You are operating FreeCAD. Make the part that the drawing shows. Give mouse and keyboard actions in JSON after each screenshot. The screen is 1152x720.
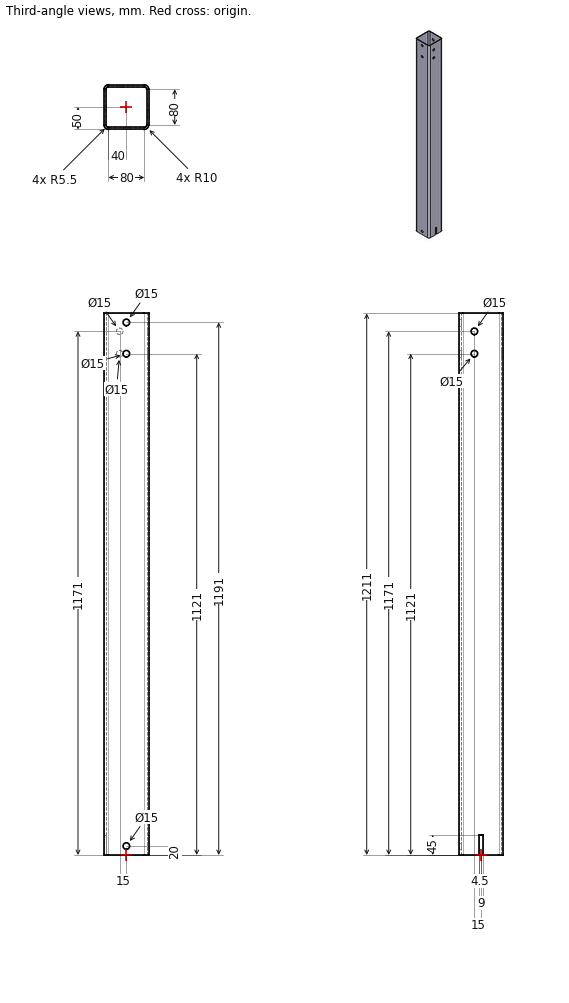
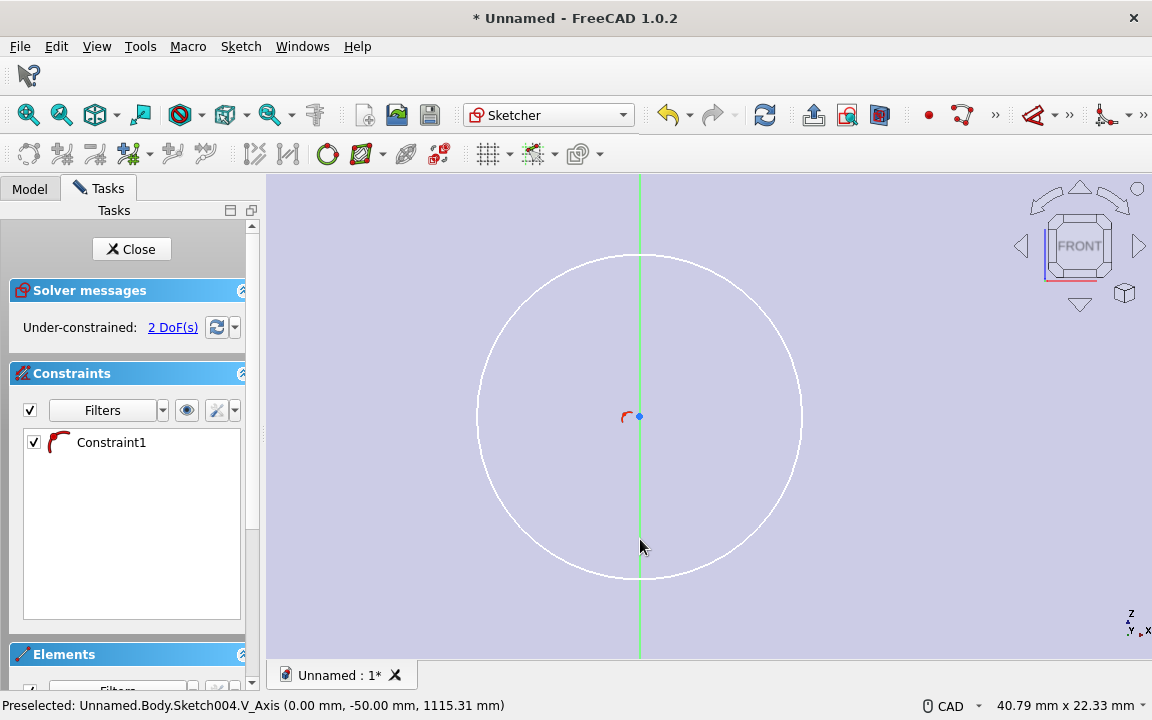
{"action": "key", "text": "d"}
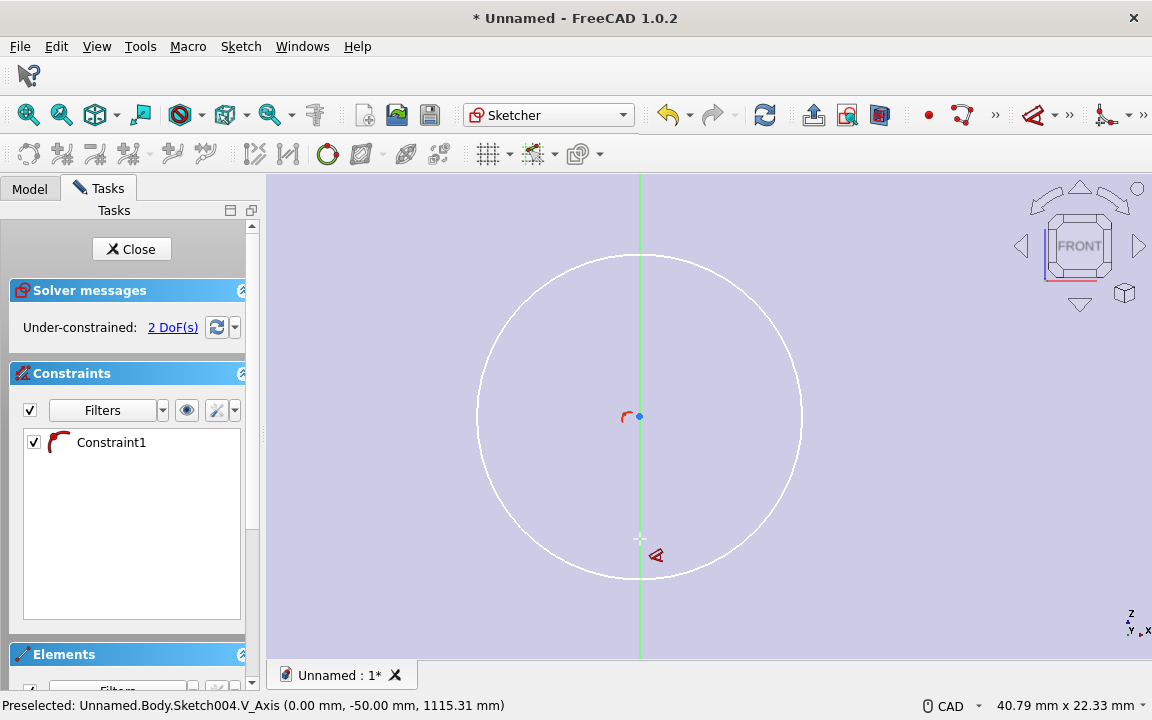
{"action": "left_click", "coordinate": [754, 302]}
{"action": "left_click", "coordinate": [777, 279]}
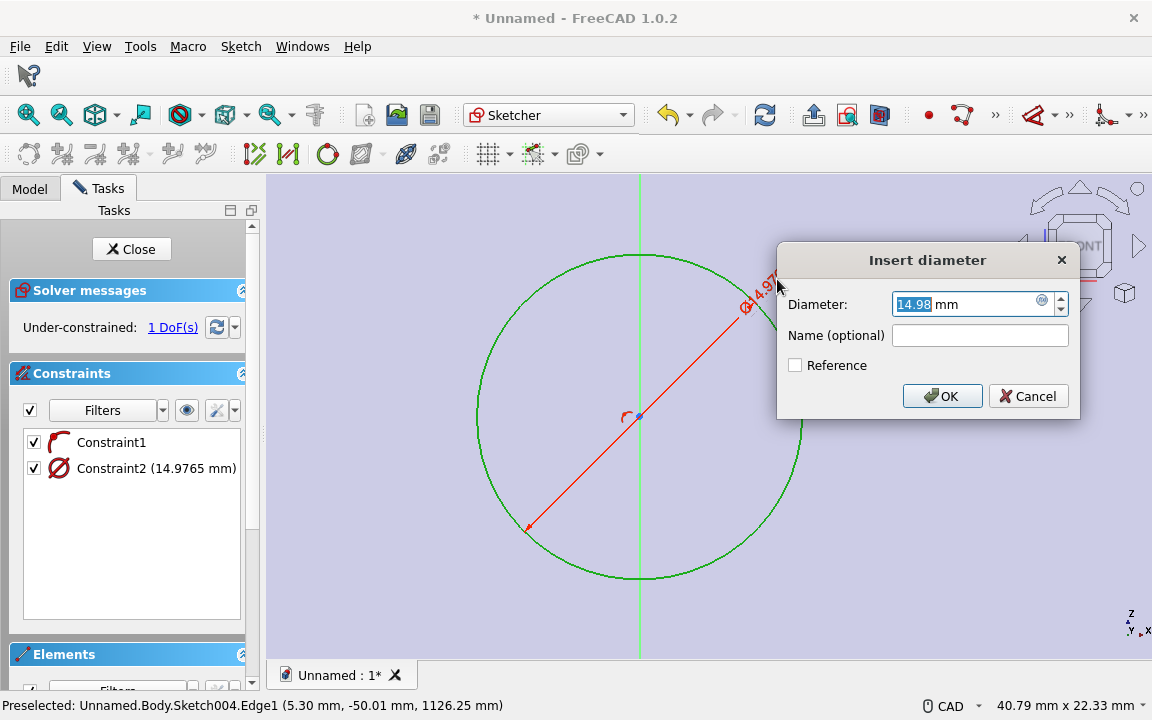
{"action": "type", "text": "15"}
{"action": "key", "text": "Return"}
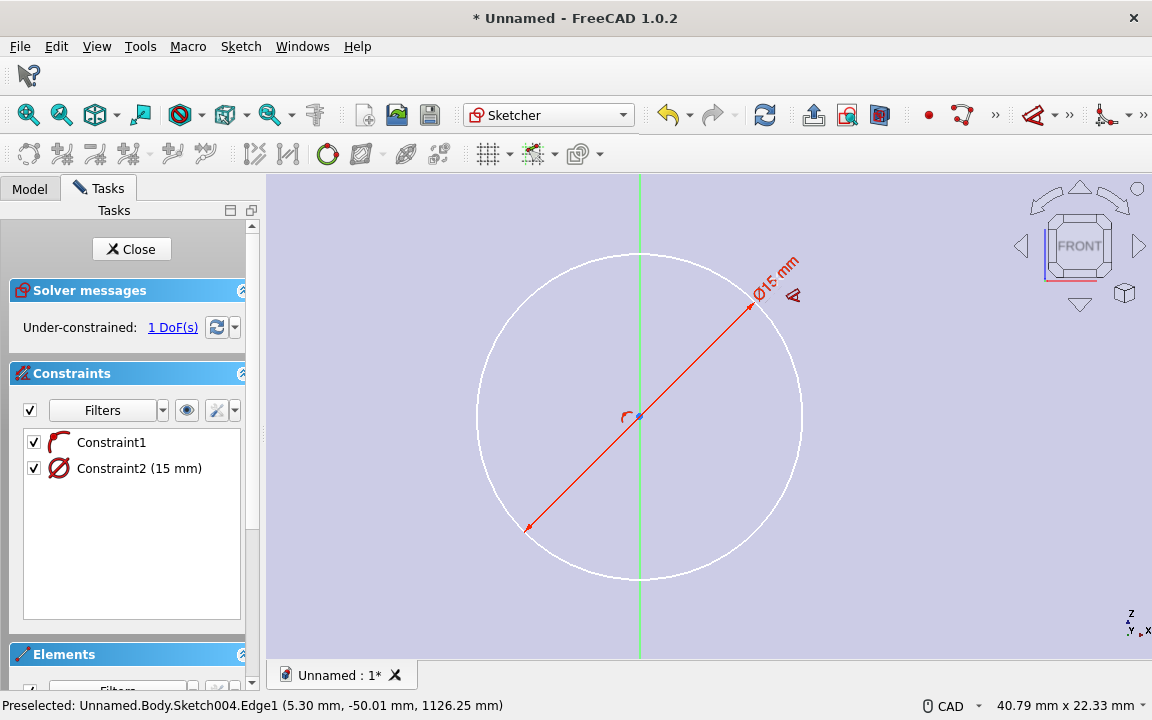
{"action": "left_click", "coordinate": [640, 417]}
{"action": "left_click", "coordinate": [674, 524]}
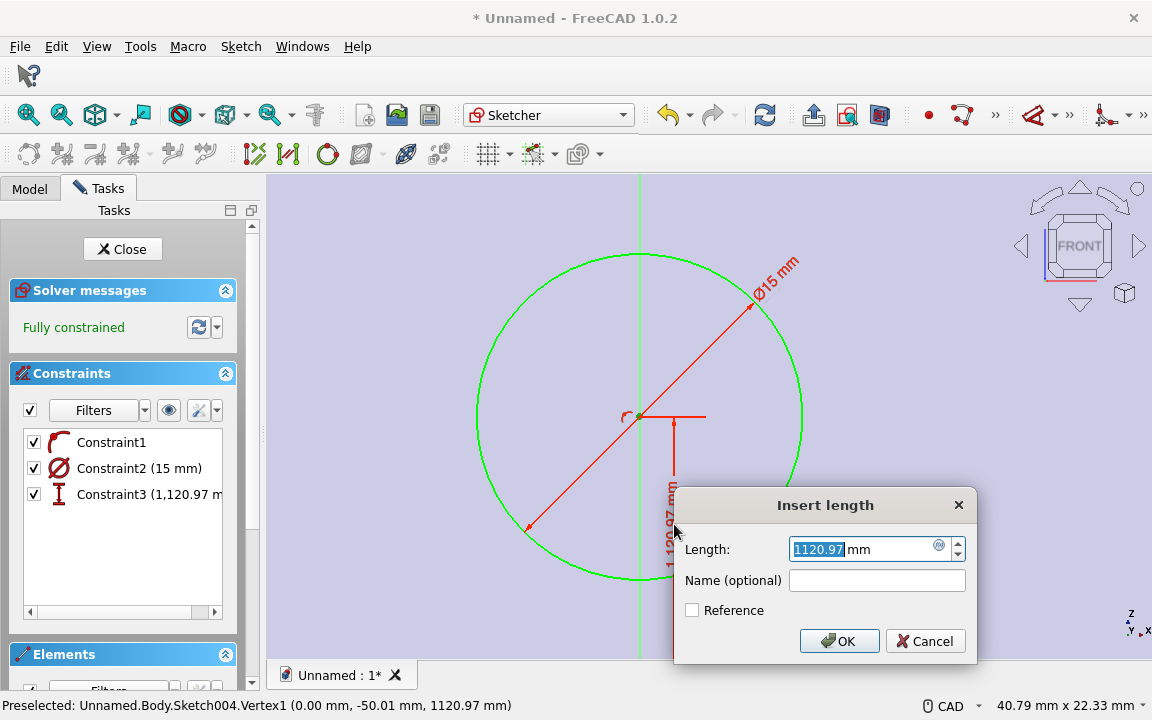
{"action": "type", "text": "1121"}
{"action": "key", "text": "Return"}
{"action": "key", "text": "Escape"}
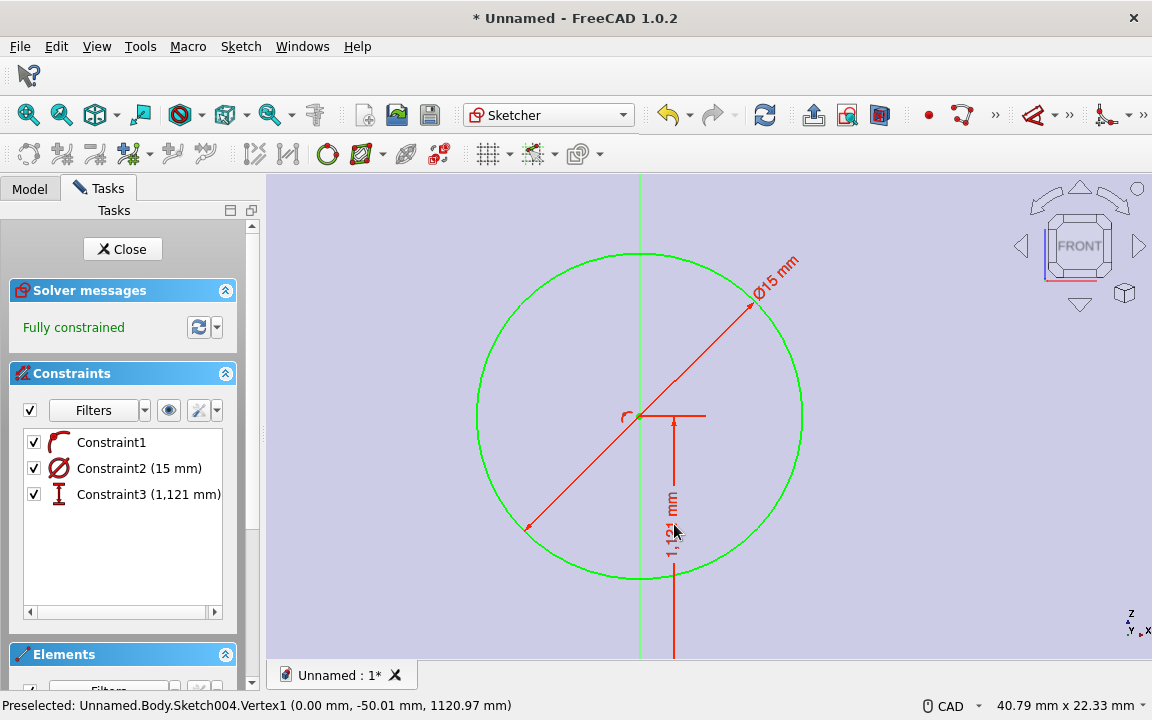
{"action": "left_click", "coordinate": [123, 249]}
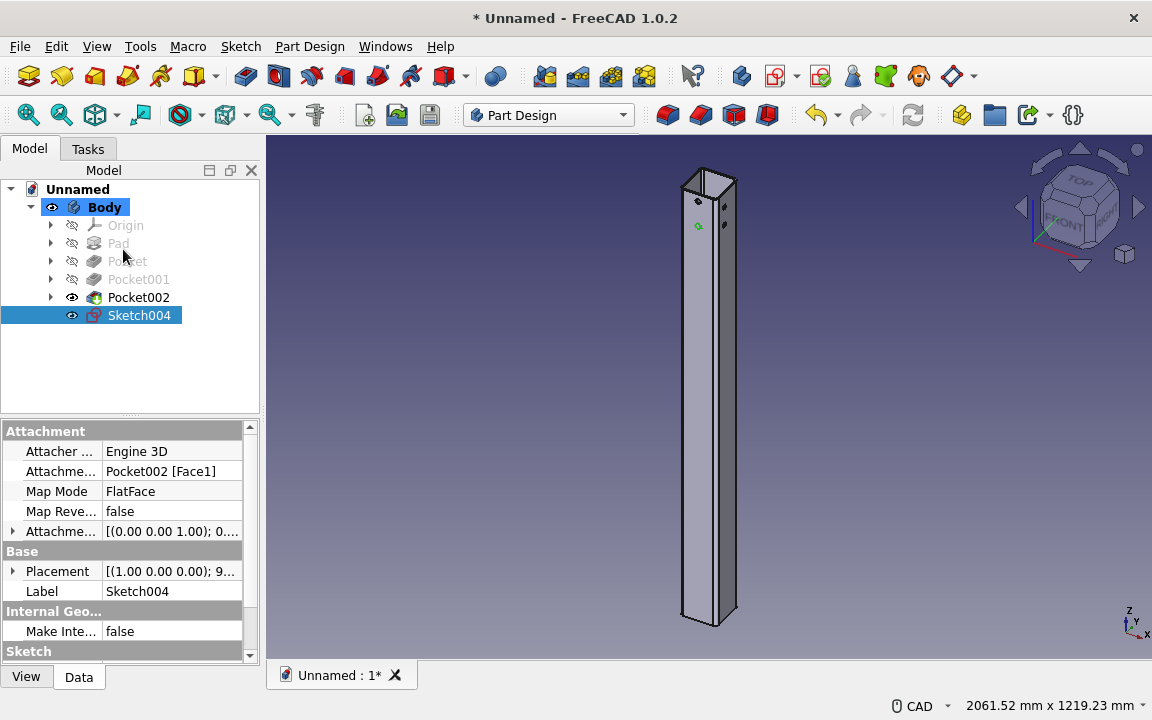
{"action": "left_click", "coordinate": [246, 76]}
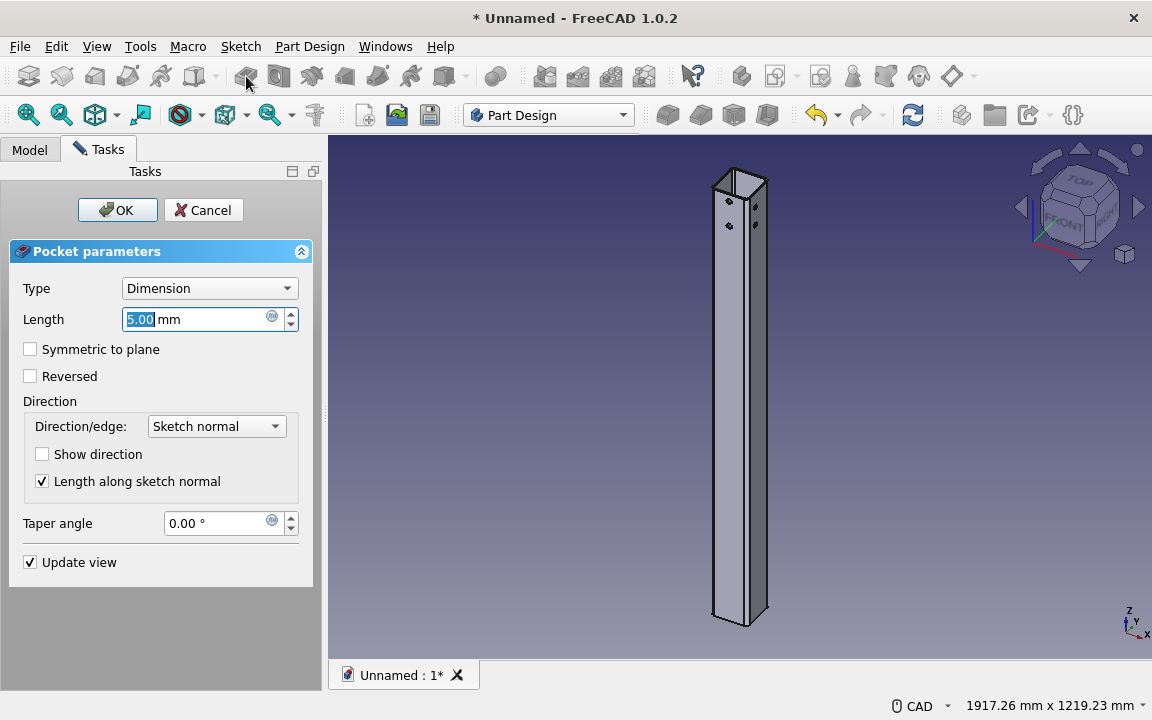
{"action": "left_click", "coordinate": [210, 288]}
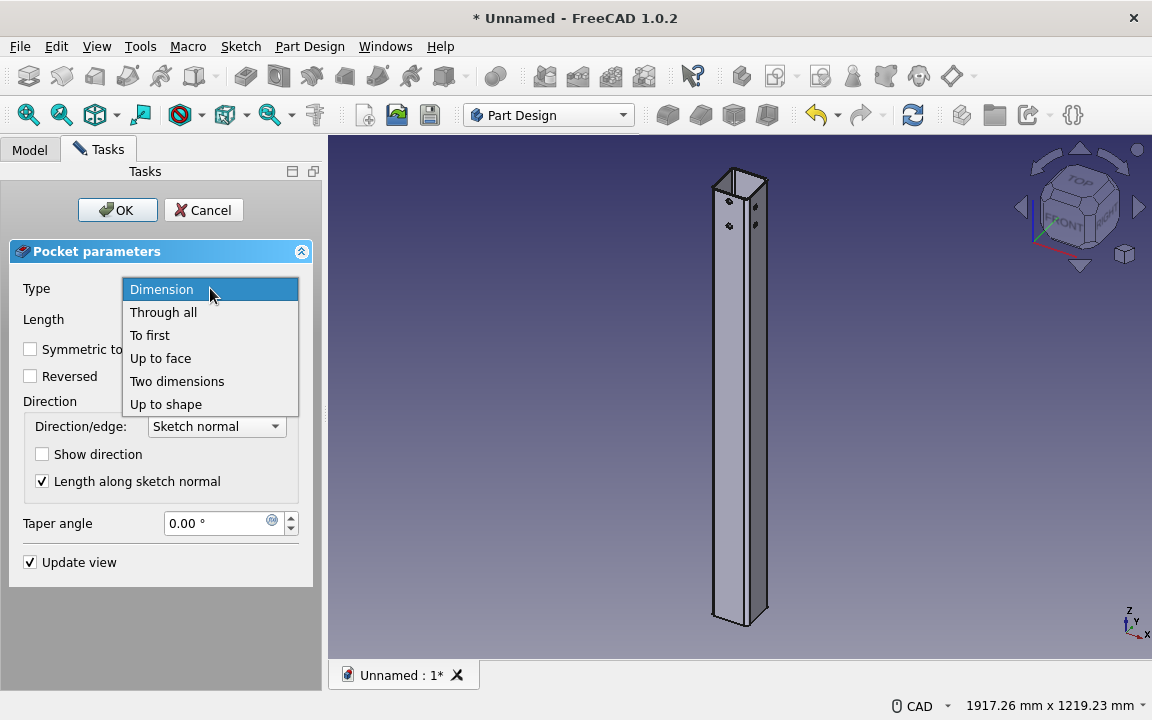
{"action": "left_click", "coordinate": [208, 336]}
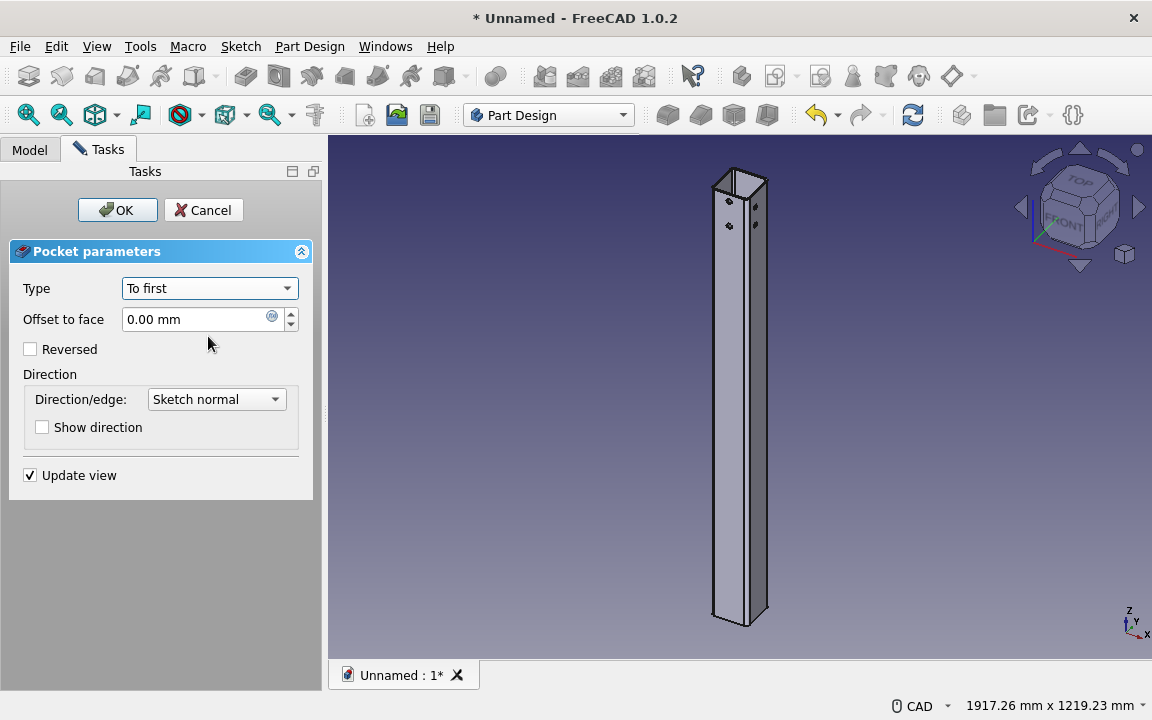
{"action": "left_click", "coordinate": [118, 210]}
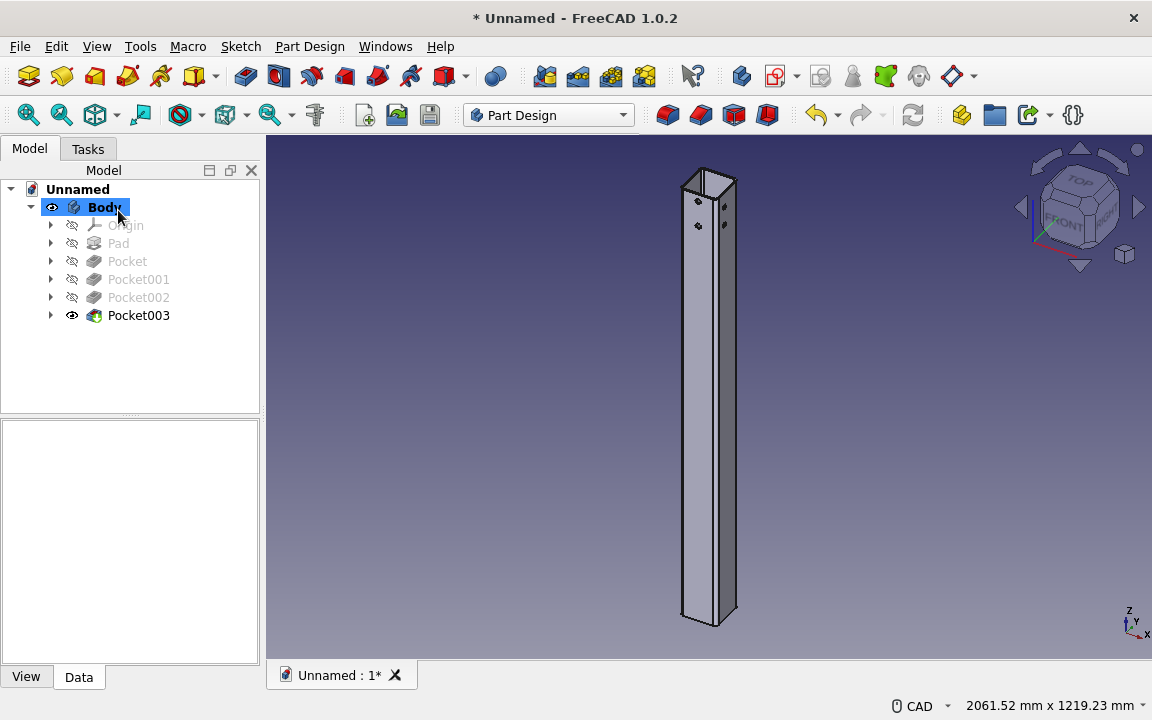
{"action": "left_click", "coordinate": [698, 285]}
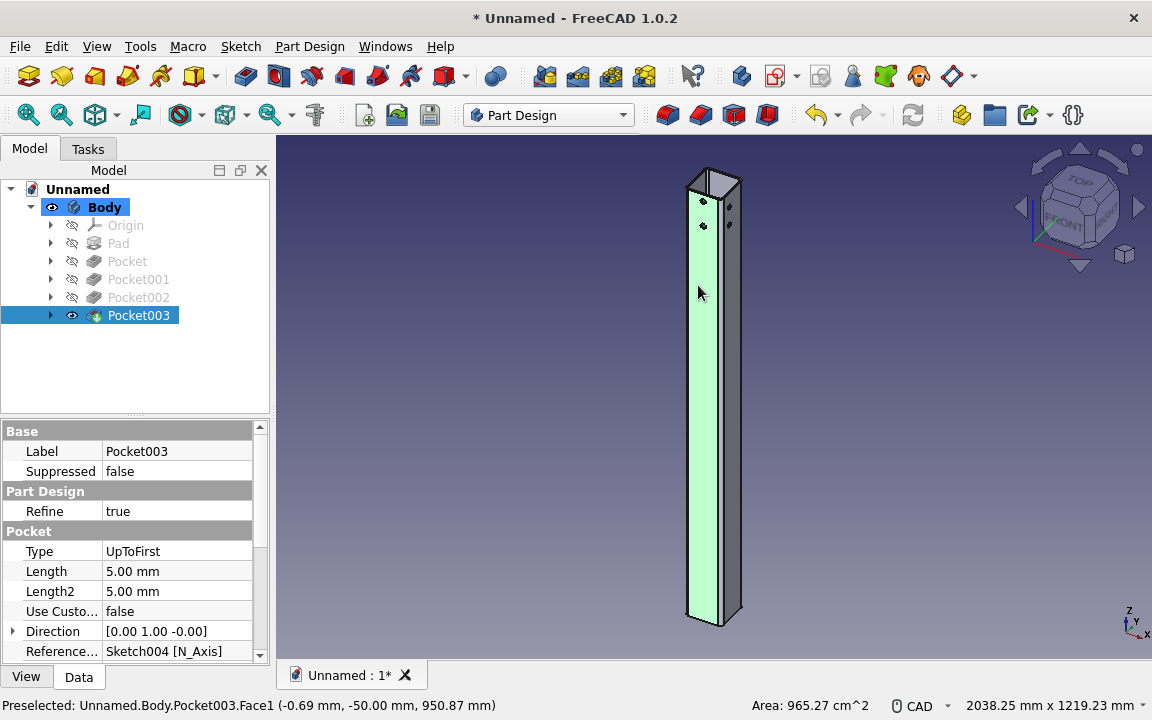
{"action": "left_click", "coordinate": [774, 76]}